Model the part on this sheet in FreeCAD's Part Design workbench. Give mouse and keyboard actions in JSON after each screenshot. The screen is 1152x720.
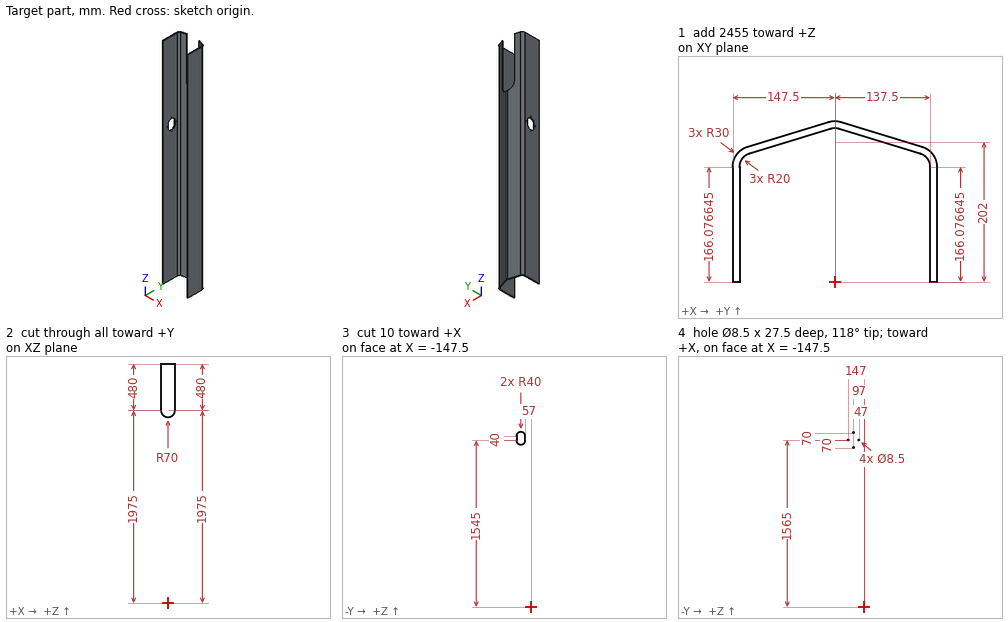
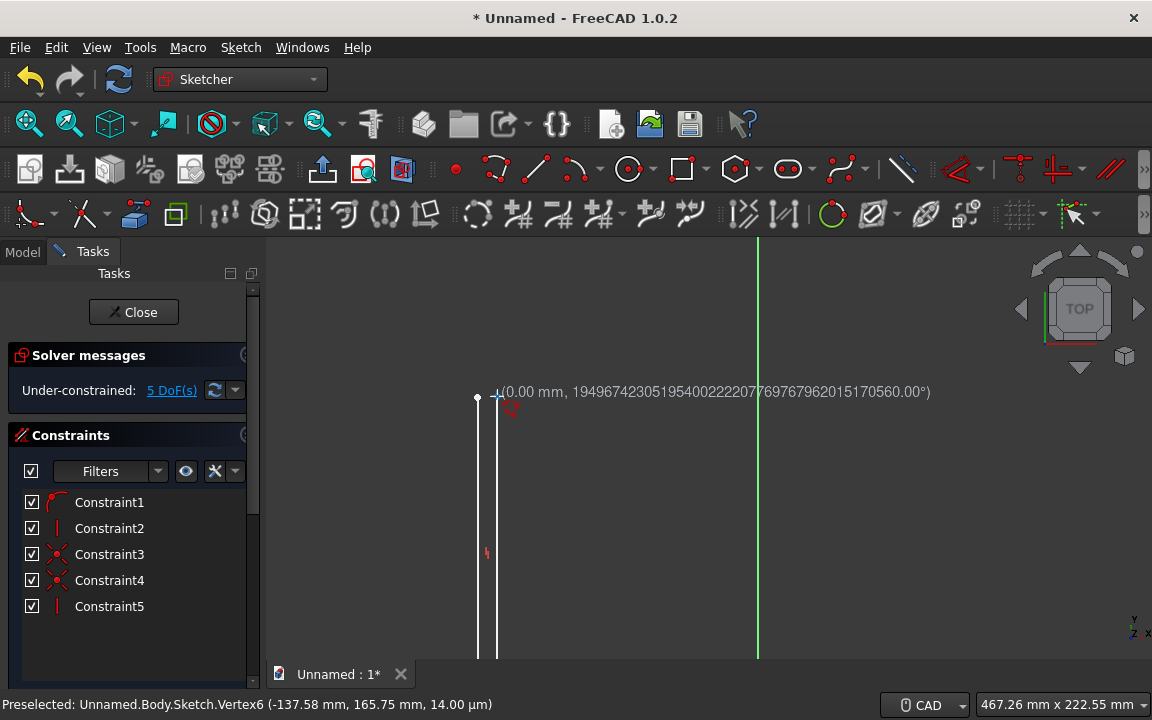
{"action": "left_click", "coordinate": [536, 170]}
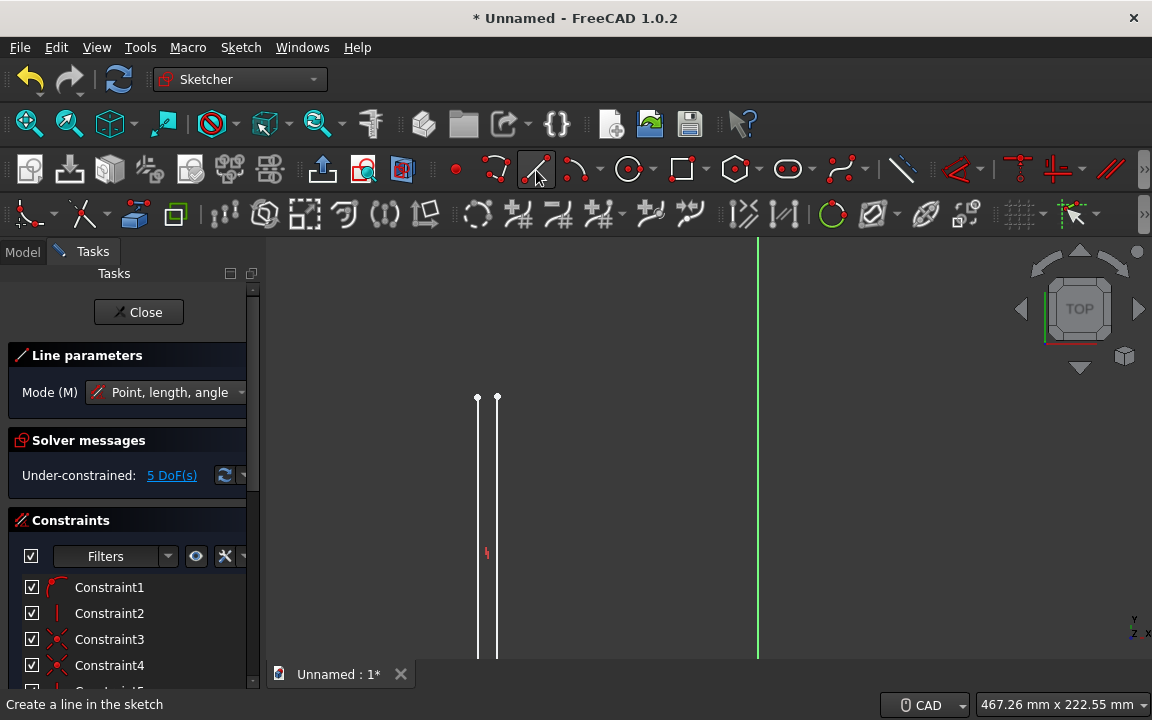
{"action": "left_click", "coordinate": [524, 360]}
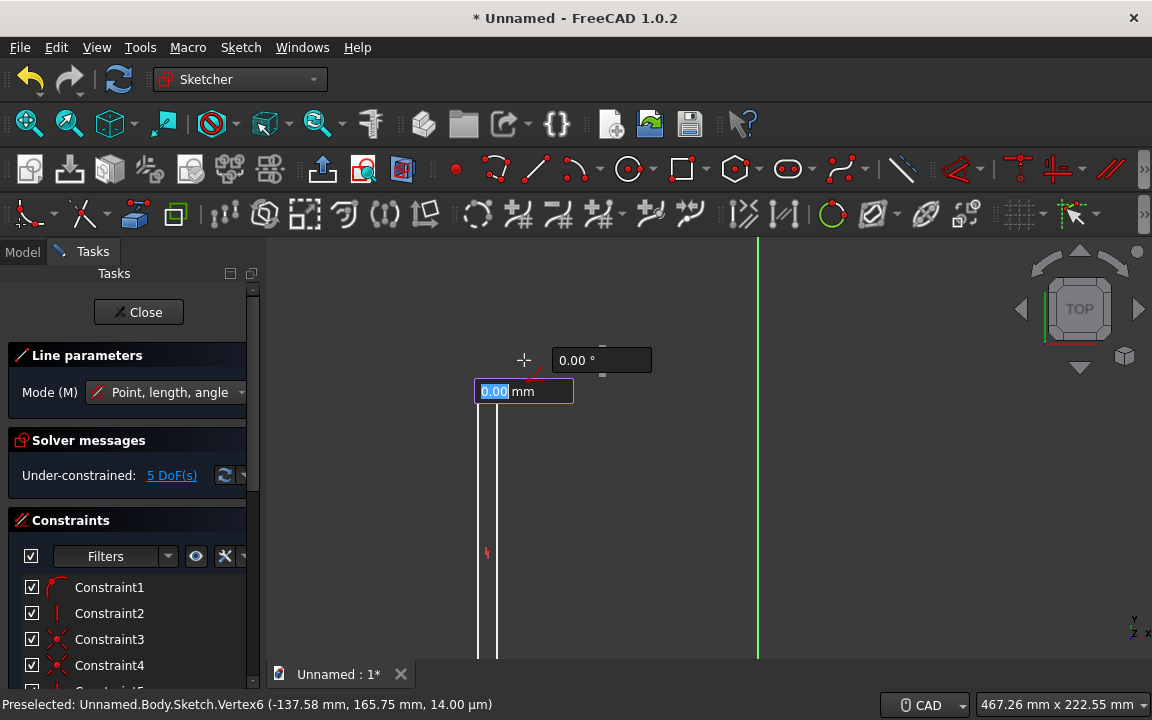
{"action": "scroll", "coordinate": [747, 292], "scroll_direction": "up", "scroll_amount": 2}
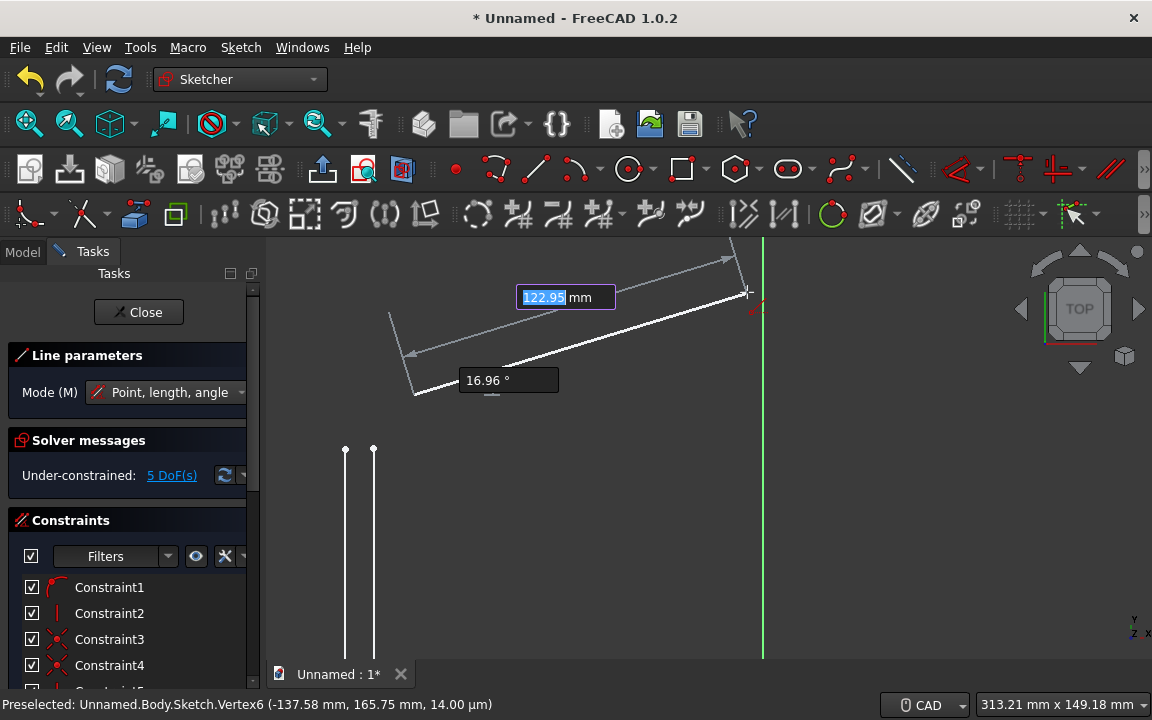
{"action": "left_click", "coordinate": [746, 292]}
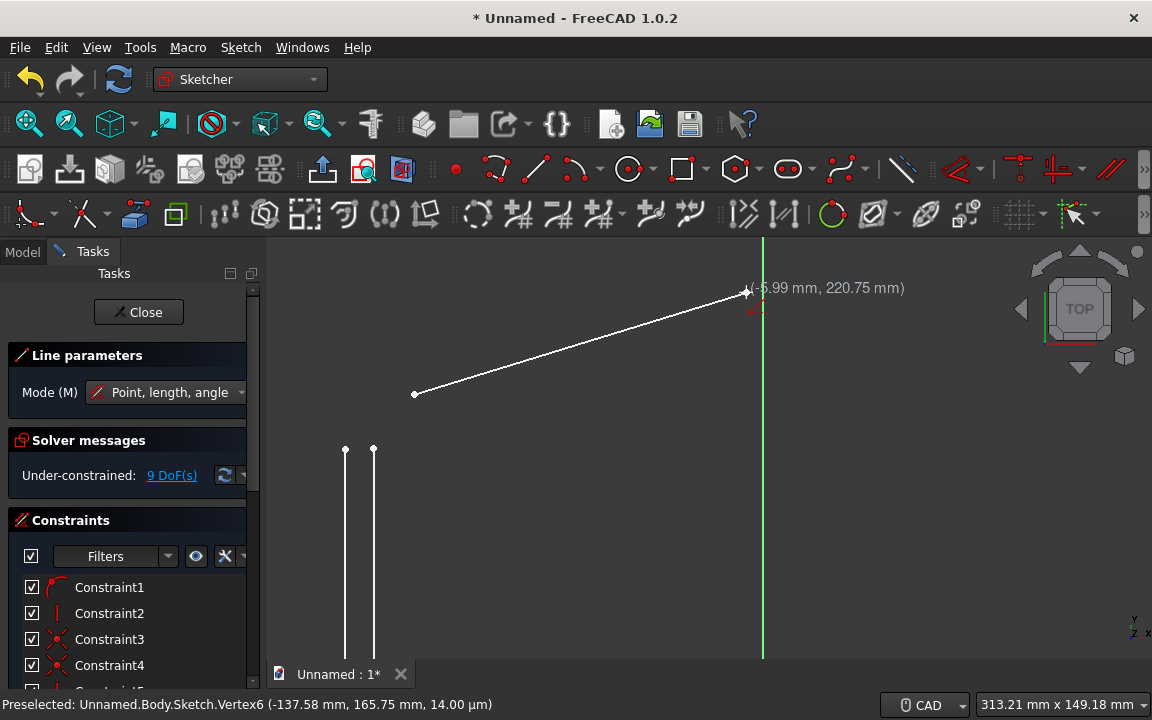
{"action": "left_click", "coordinate": [779, 292]}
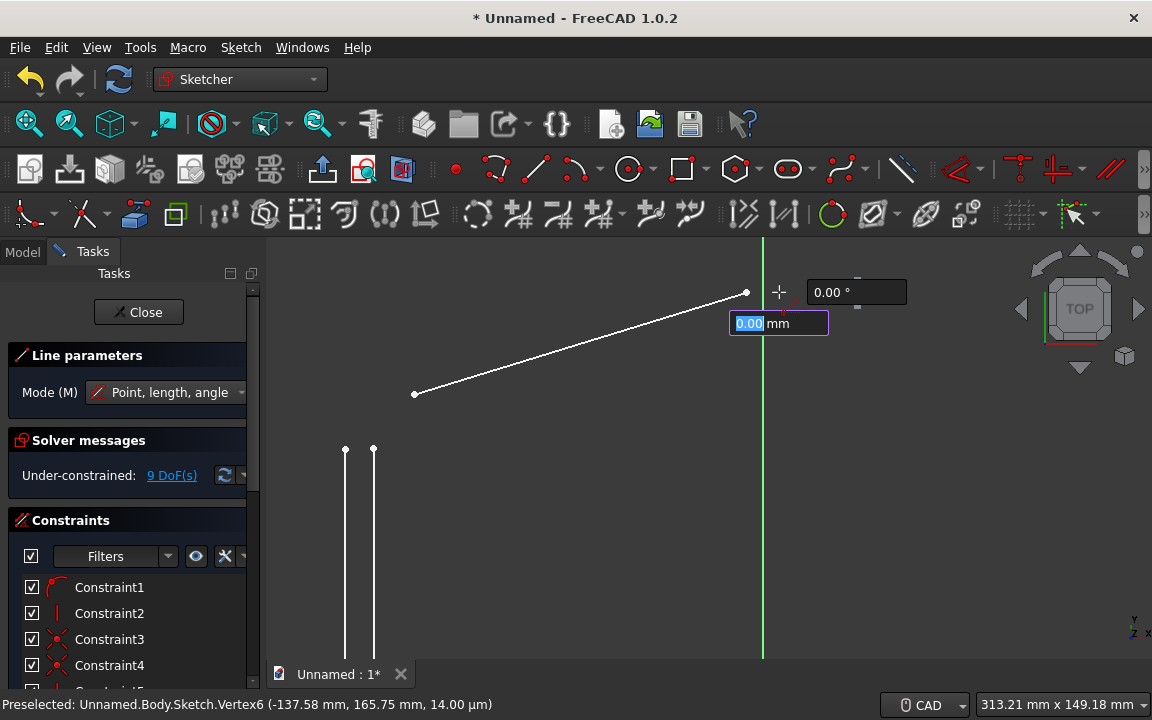
{"action": "scroll", "coordinate": [569, 366], "scroll_direction": "down", "scroll_amount": 5}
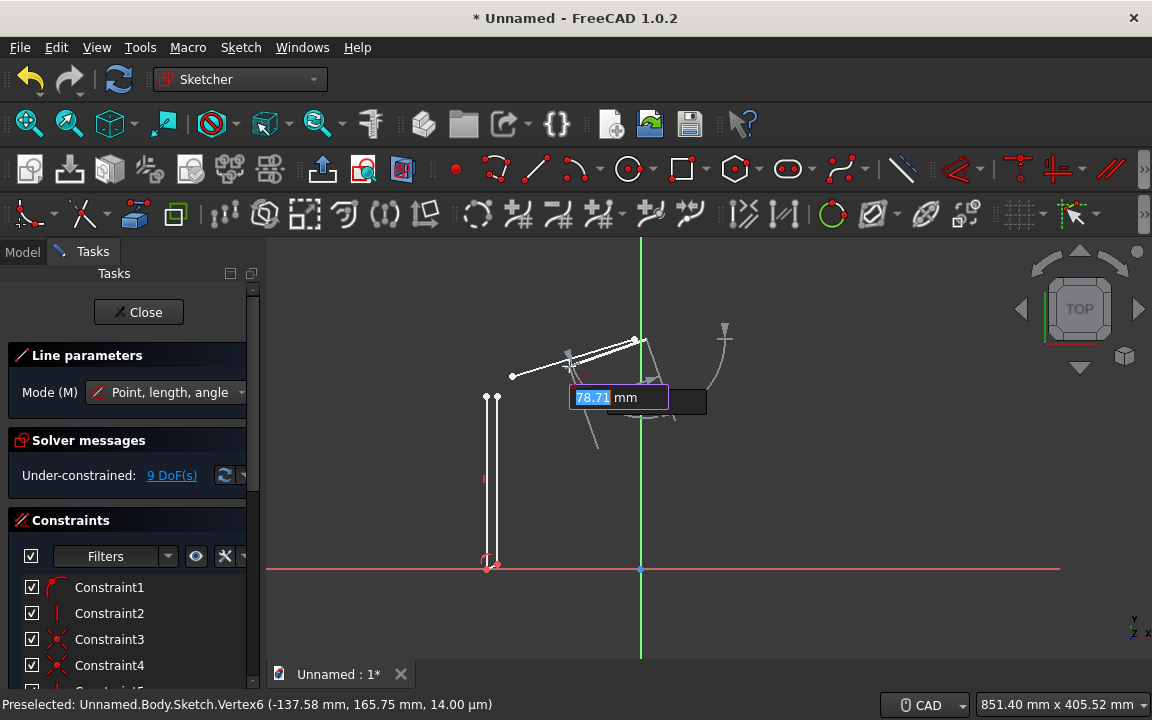
{"action": "left_click", "coordinate": [769, 376]}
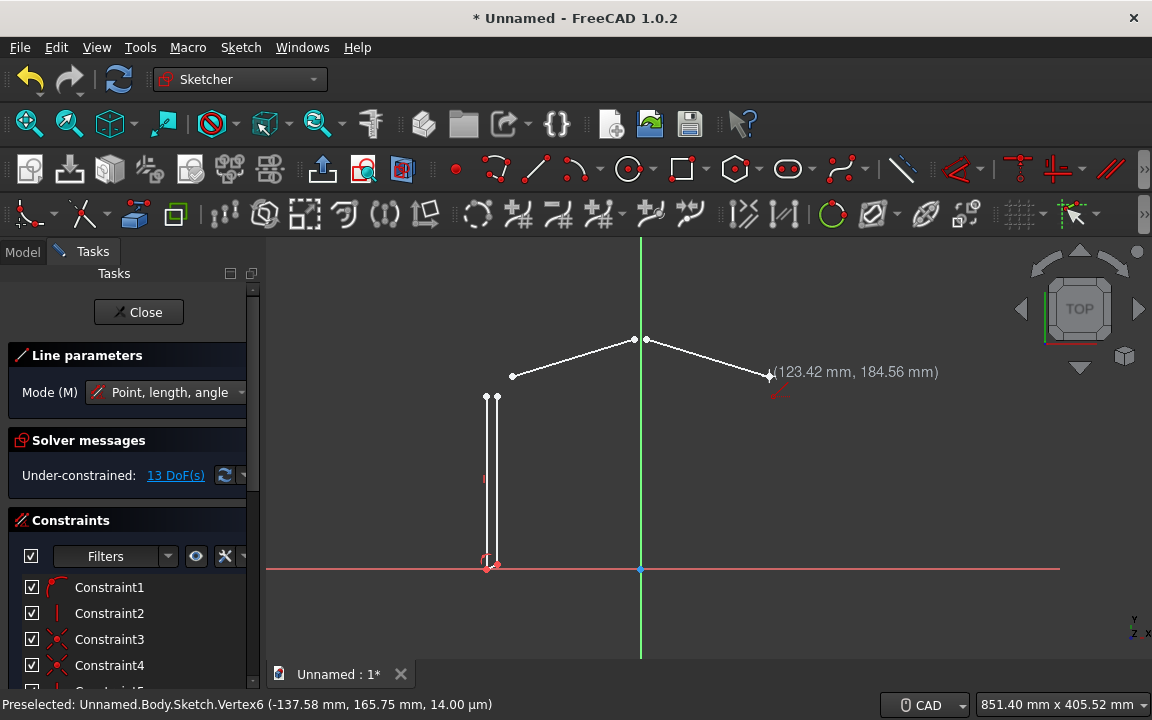
{"action": "left_click", "coordinate": [496, 170]}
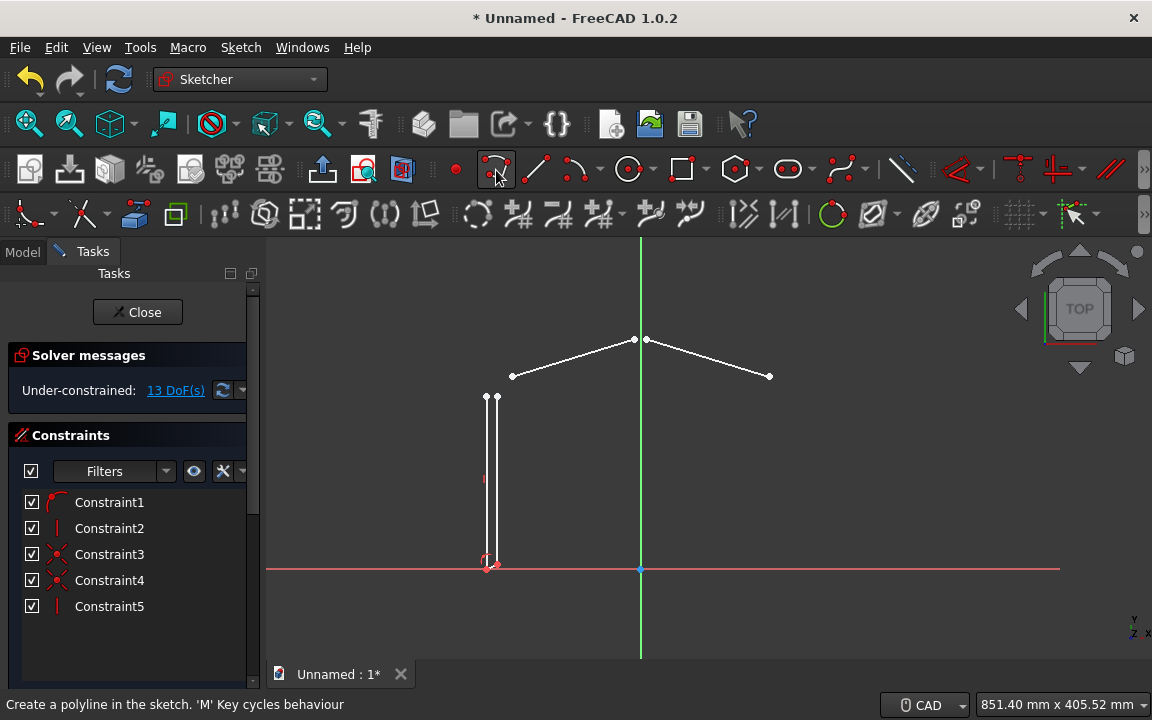
{"action": "left_click", "coordinate": [784, 396]}
{"action": "left_click", "coordinate": [784, 569]}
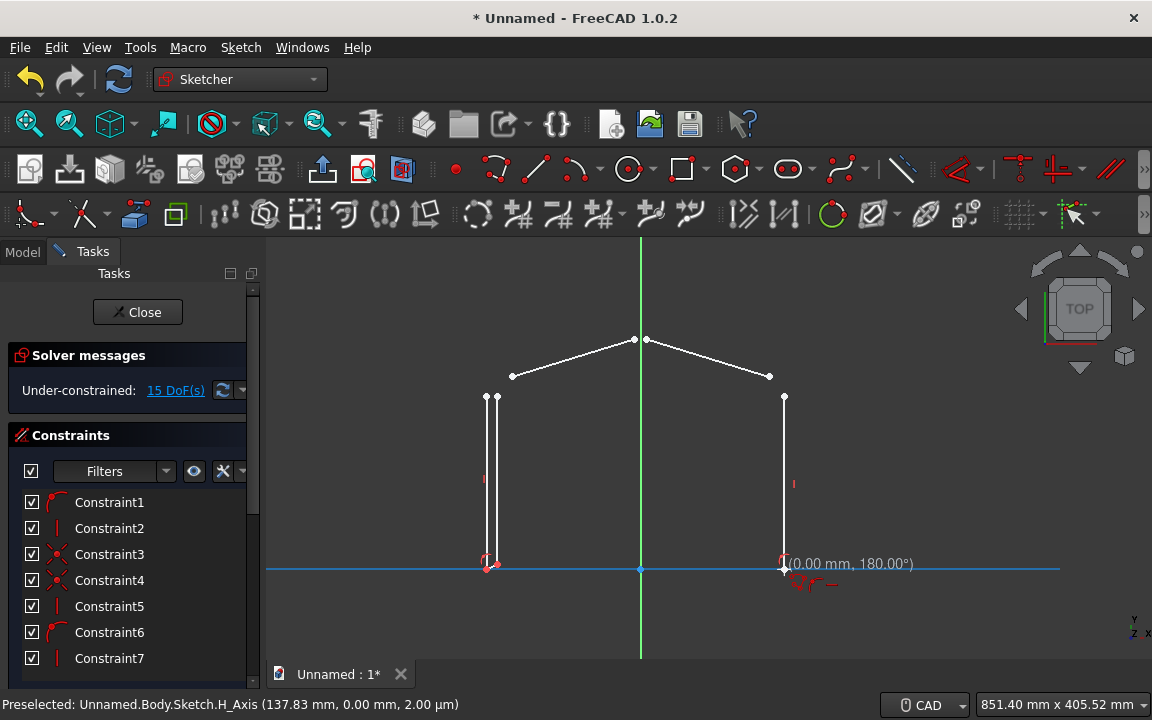
{"action": "scroll", "coordinate": [794, 569], "scroll_direction": "up", "scroll_amount": 3}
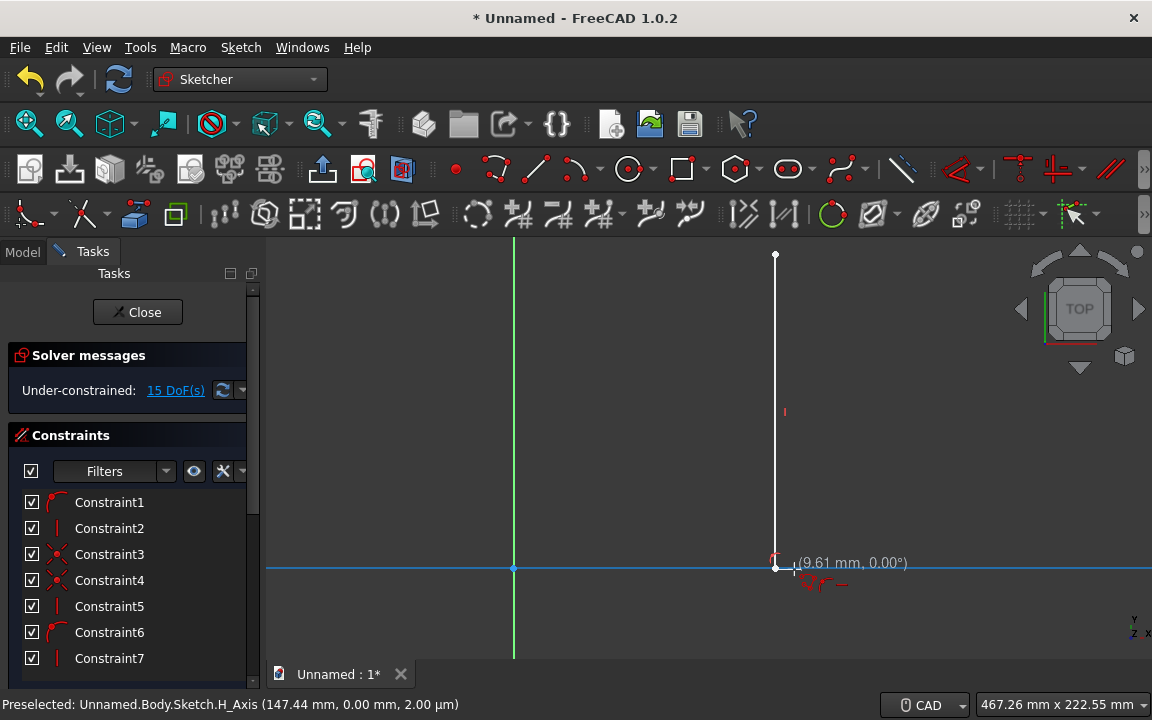
{"action": "left_click", "coordinate": [794, 559]}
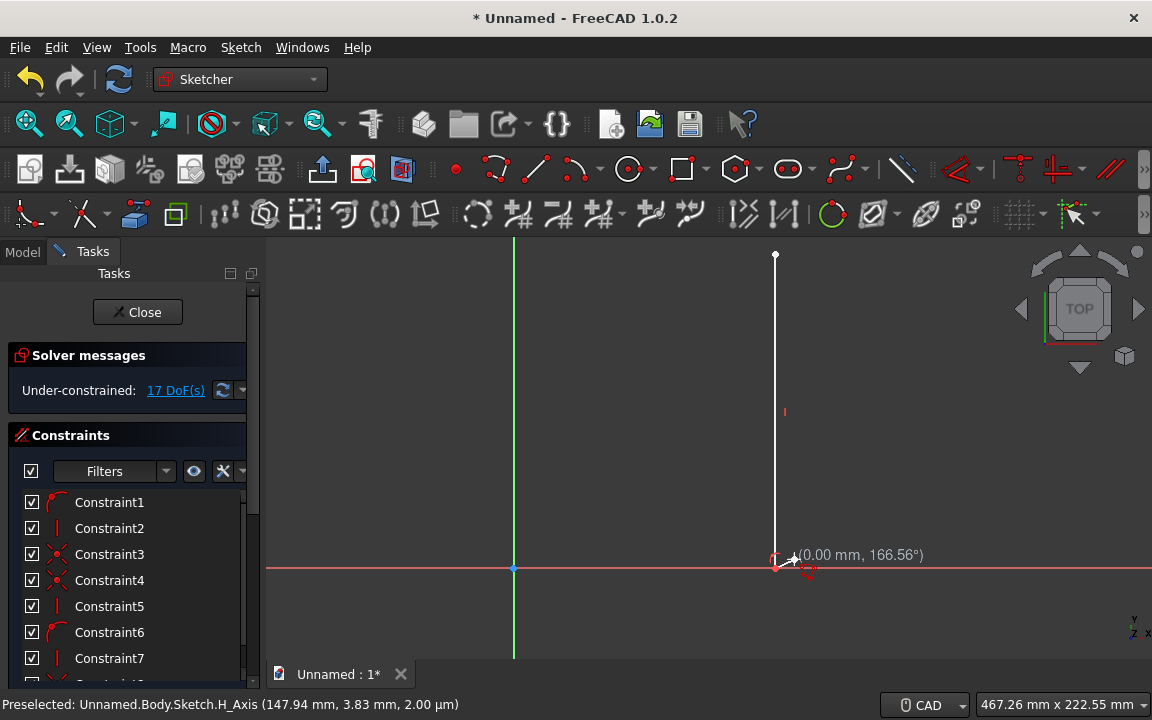
{"action": "scroll", "coordinate": [794, 569], "scroll_direction": "down", "scroll_amount": 3}